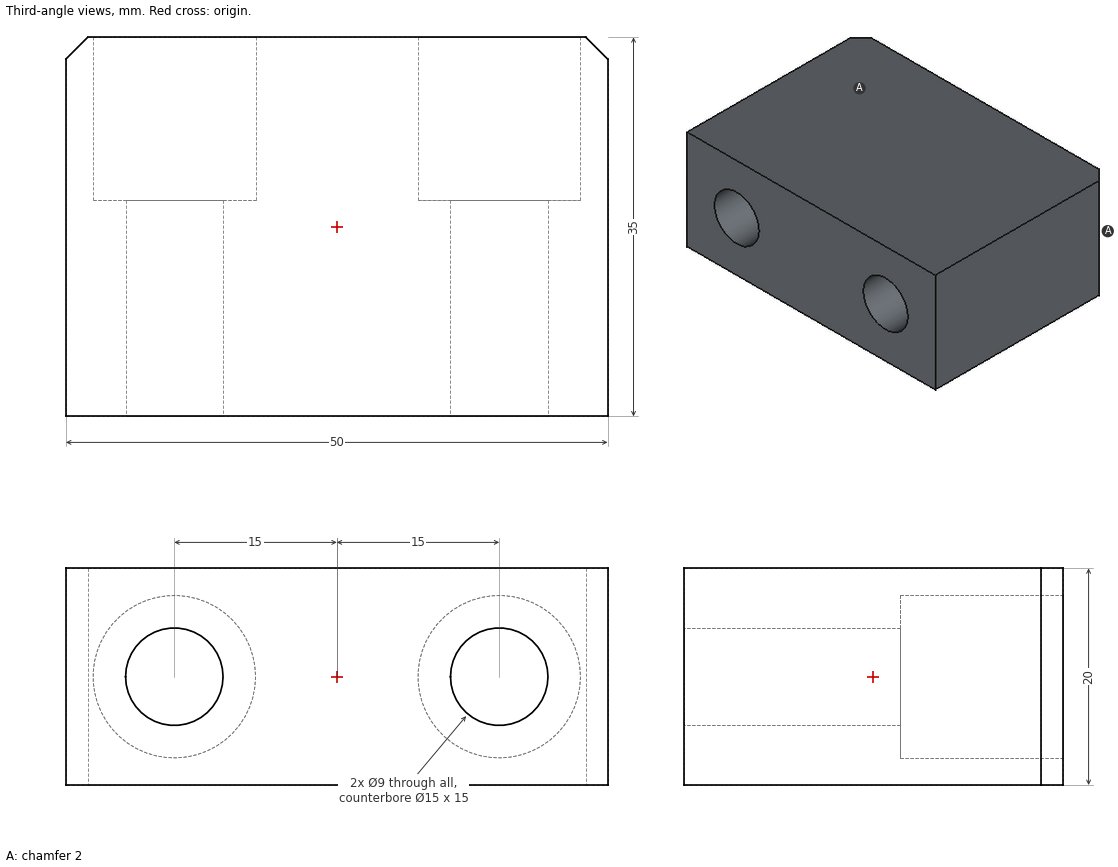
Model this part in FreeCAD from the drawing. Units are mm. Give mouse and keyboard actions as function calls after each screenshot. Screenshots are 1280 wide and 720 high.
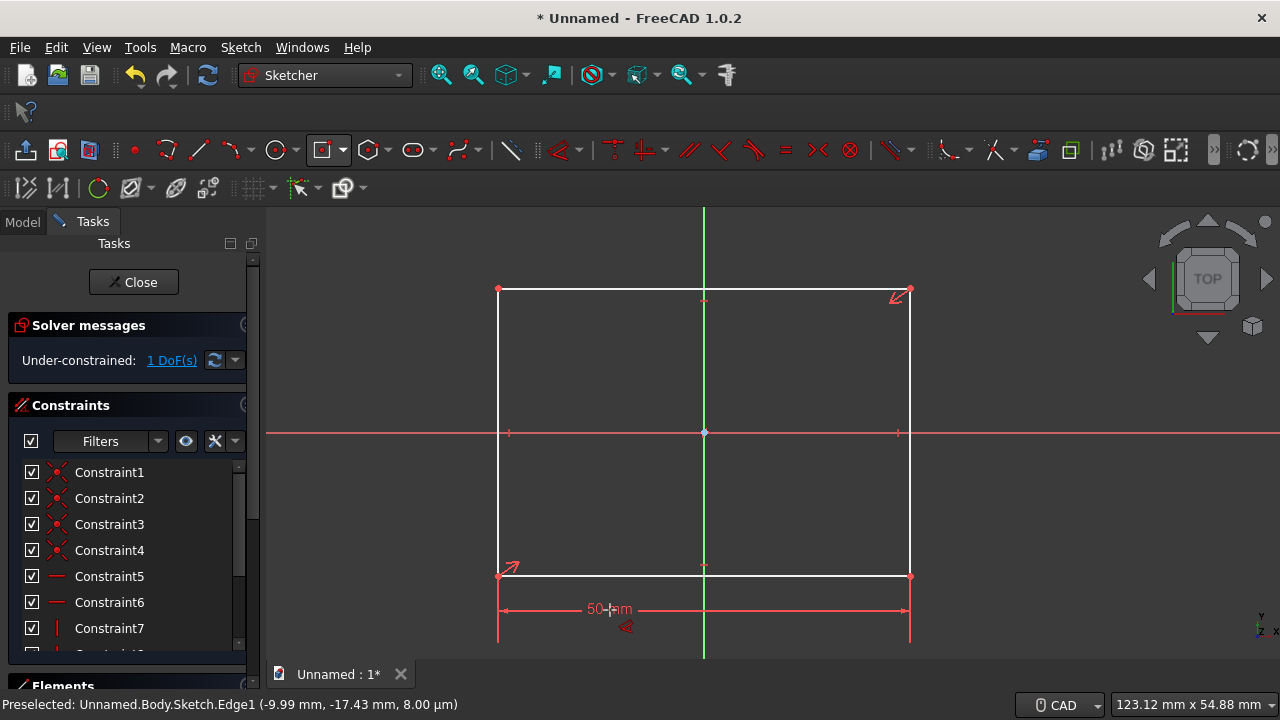
click(910, 490)
click(944, 367)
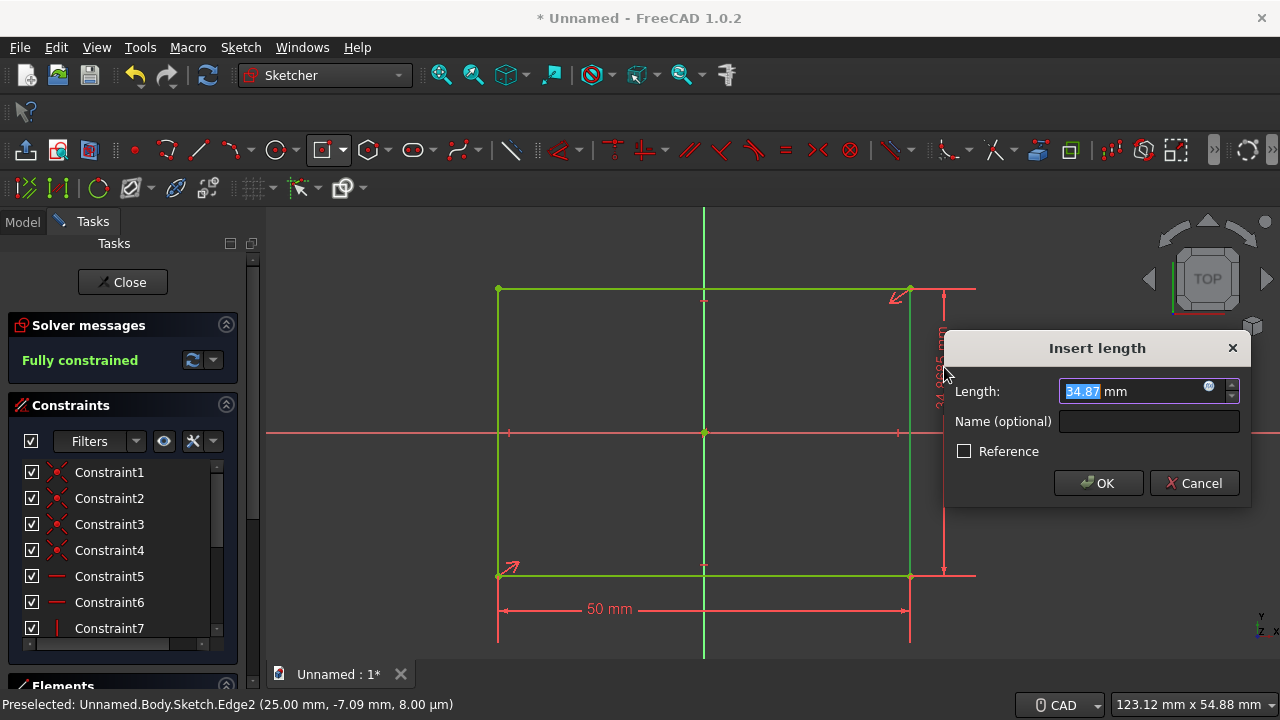
text(35)
key(Return)
key(Escape)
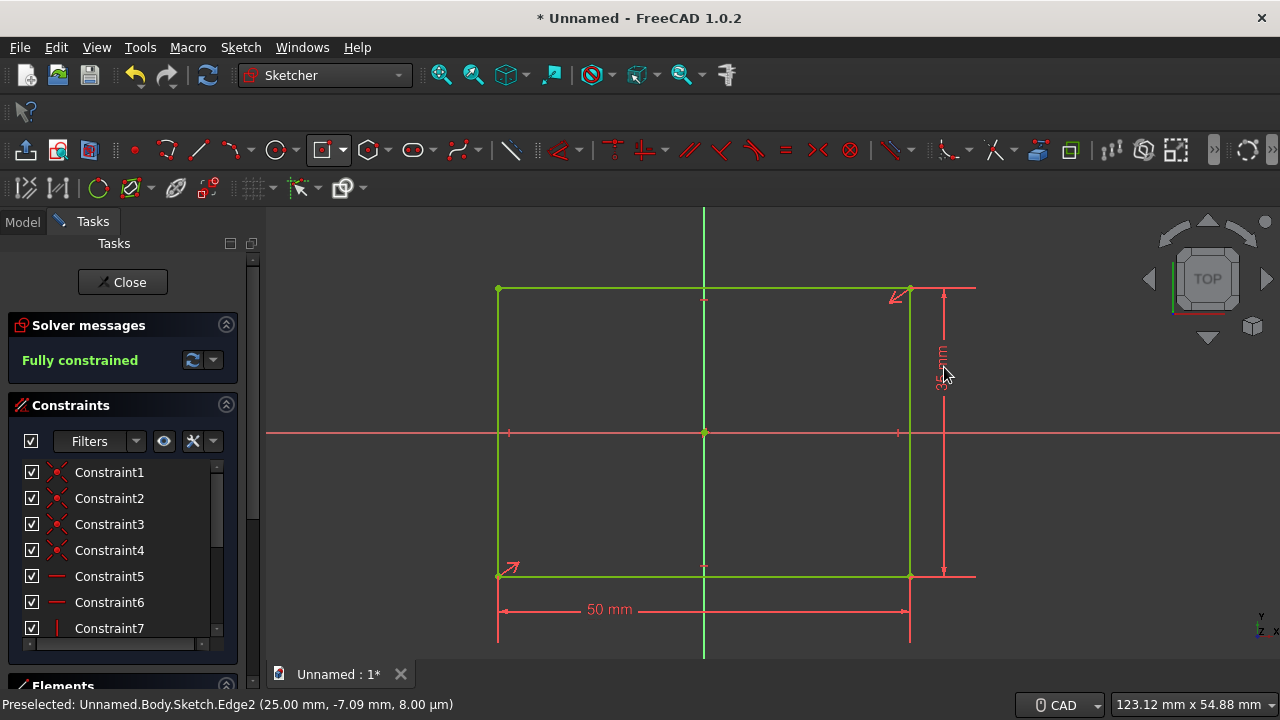
click(123, 282)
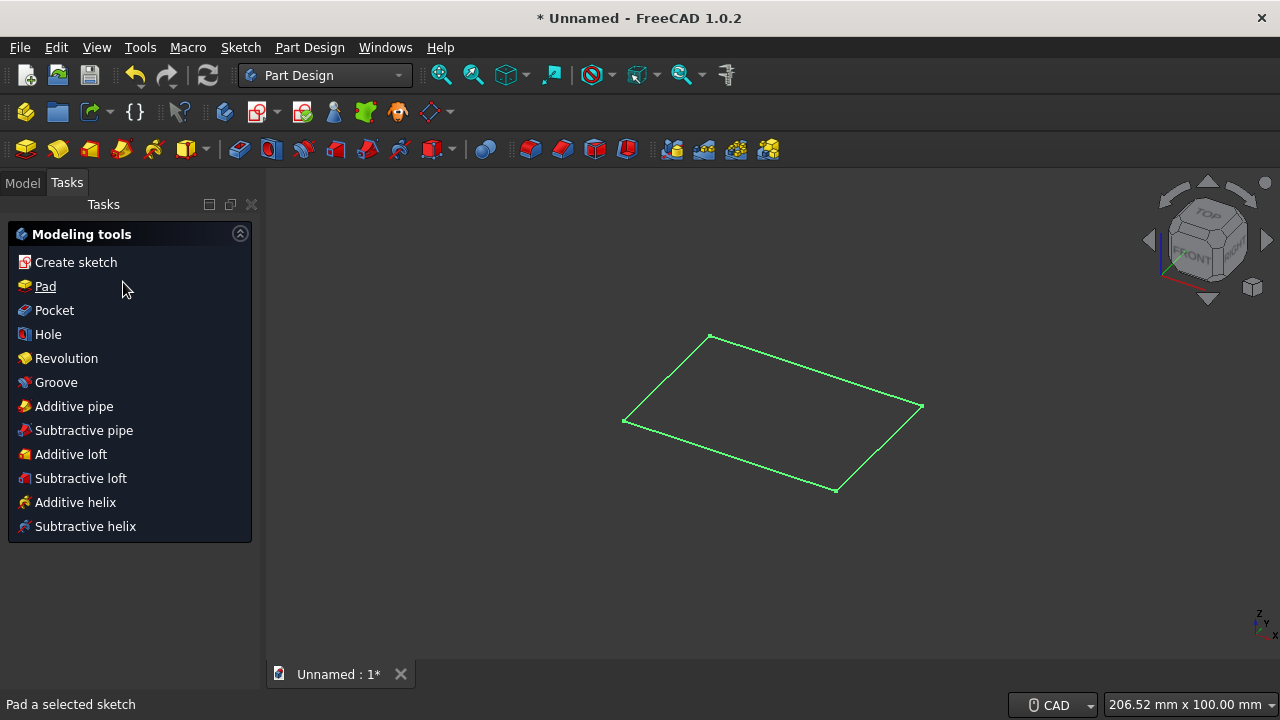
click(26, 150)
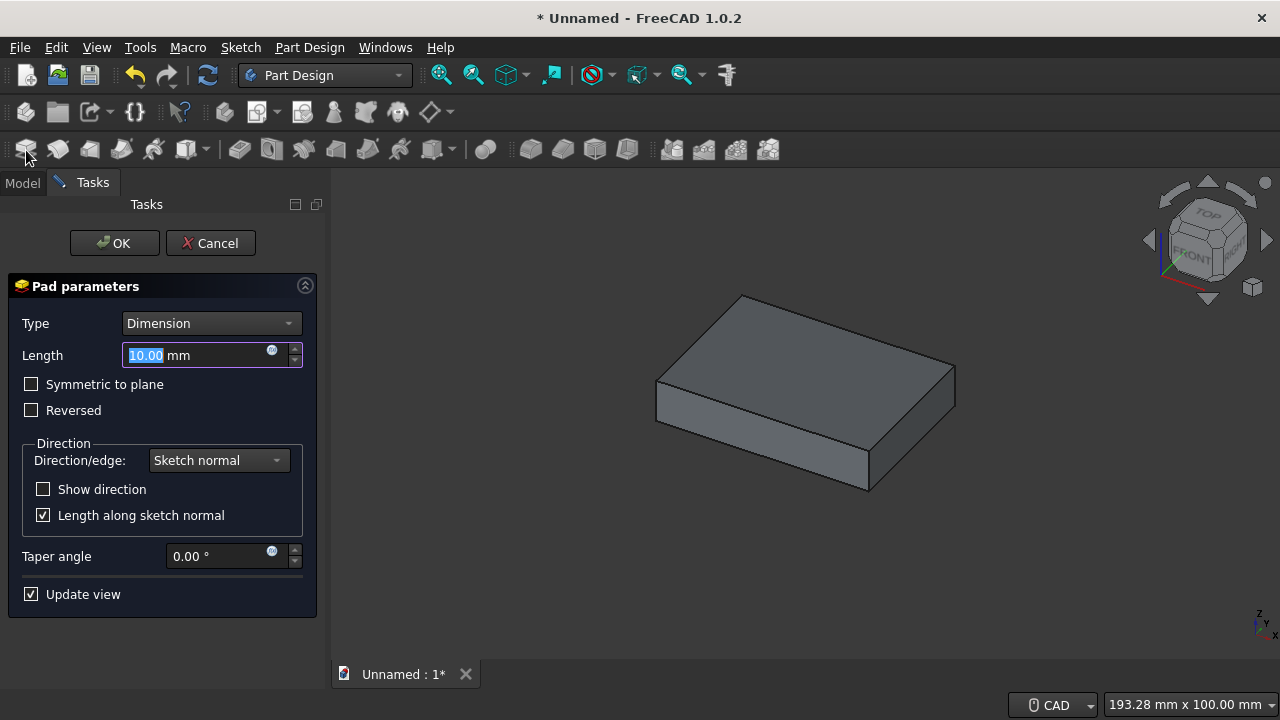
text(20)
key(Tab)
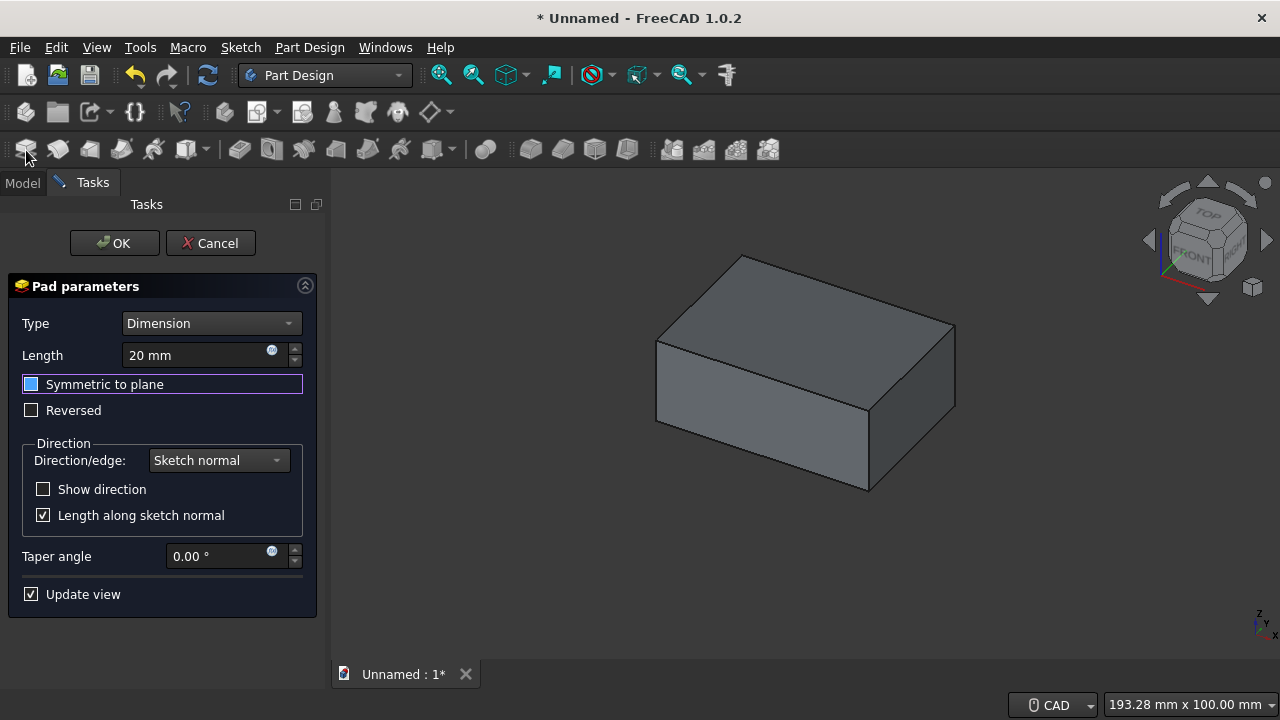
click(30, 384)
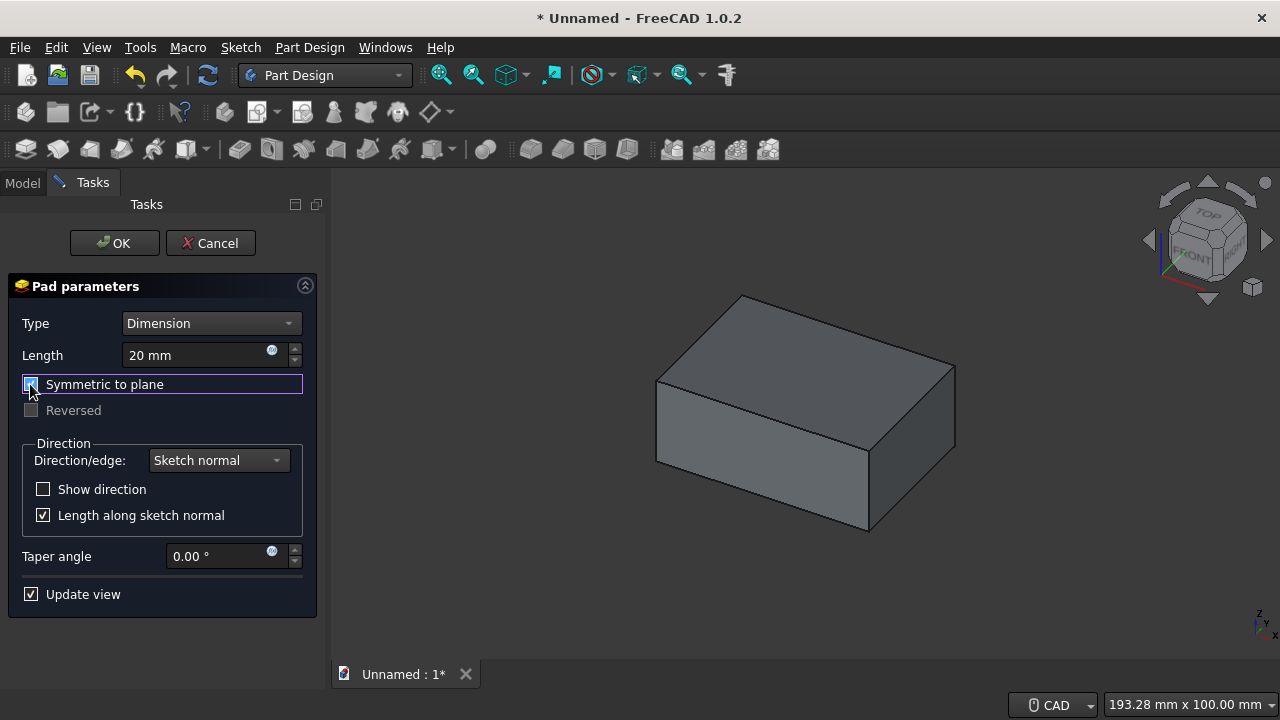
click(115, 243)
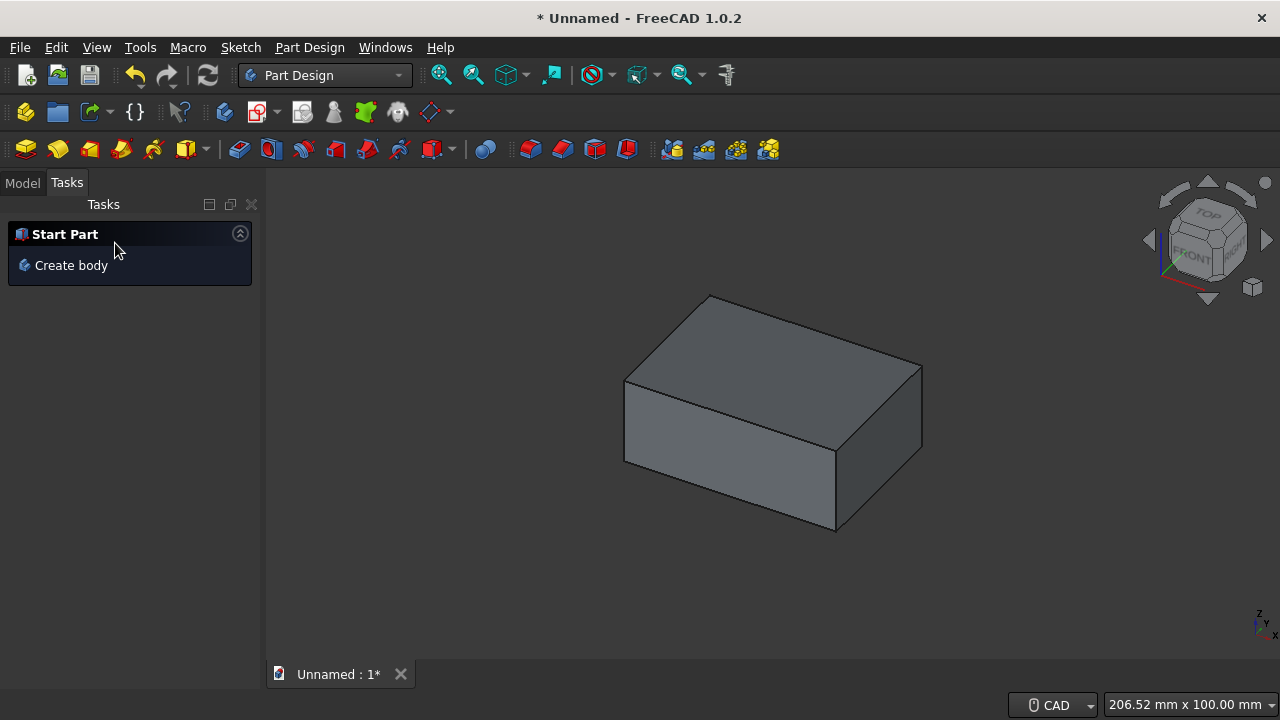
key(4)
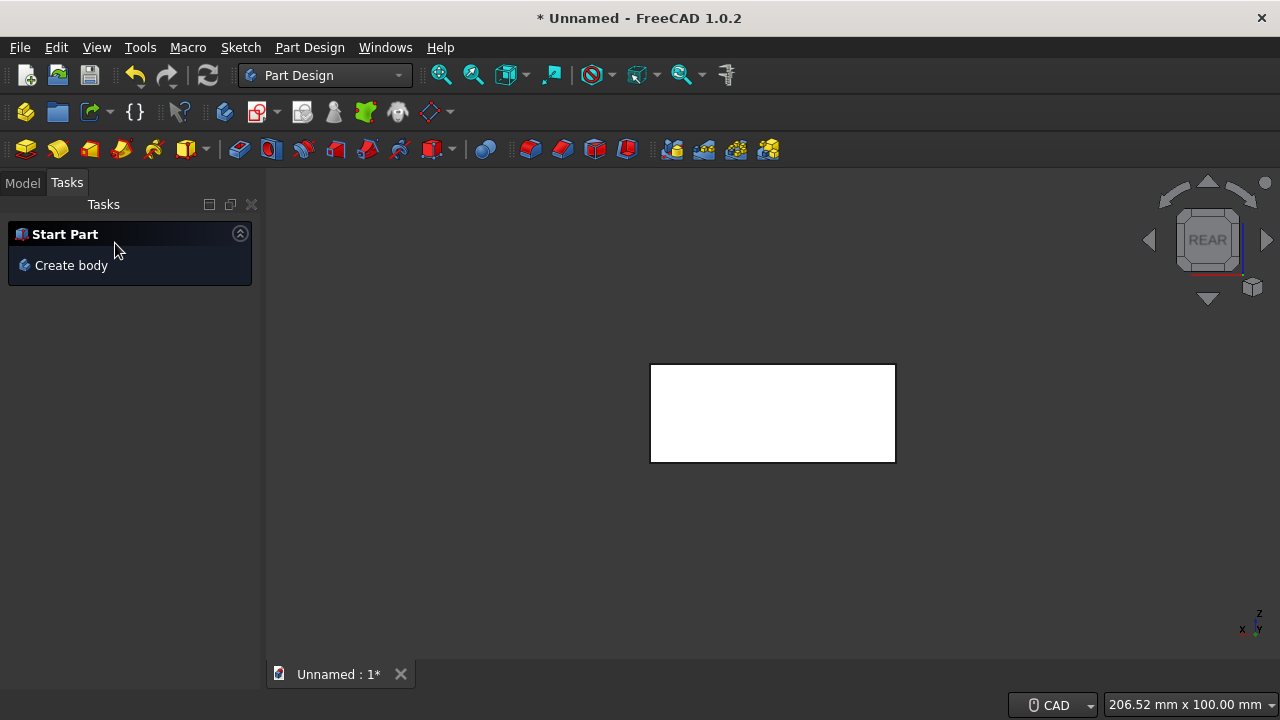
click(442, 76)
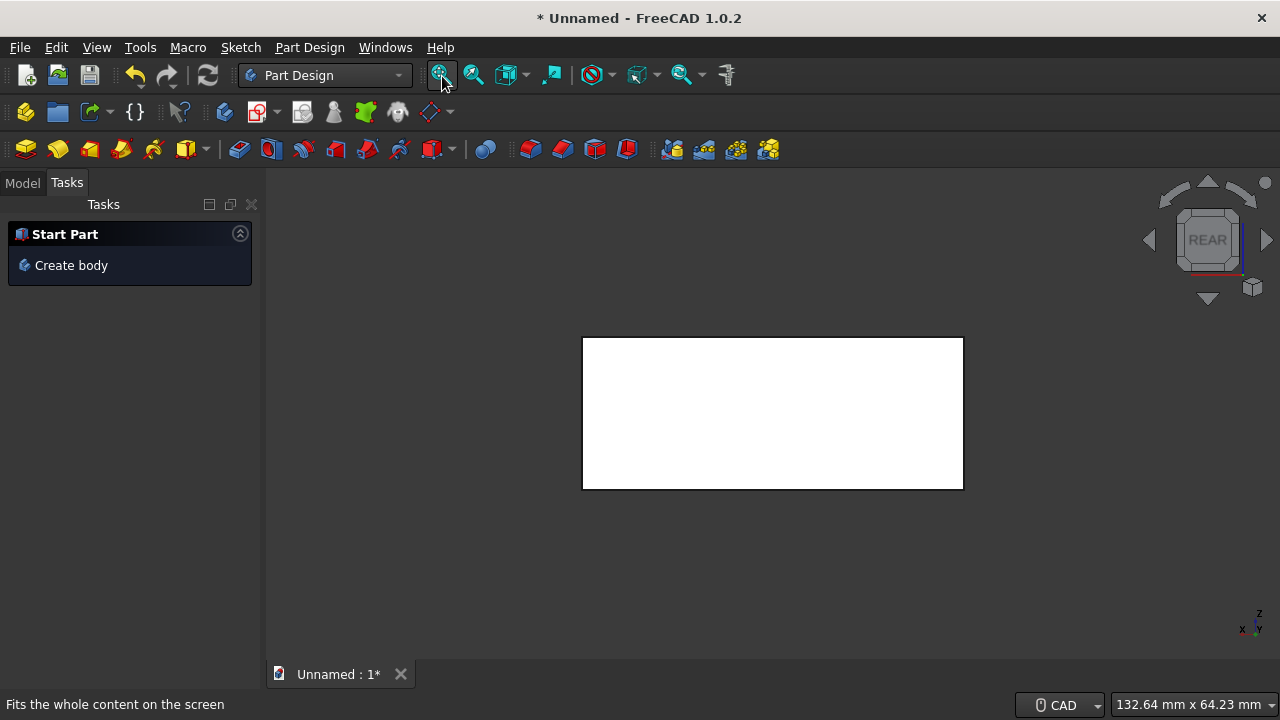
click(664, 413)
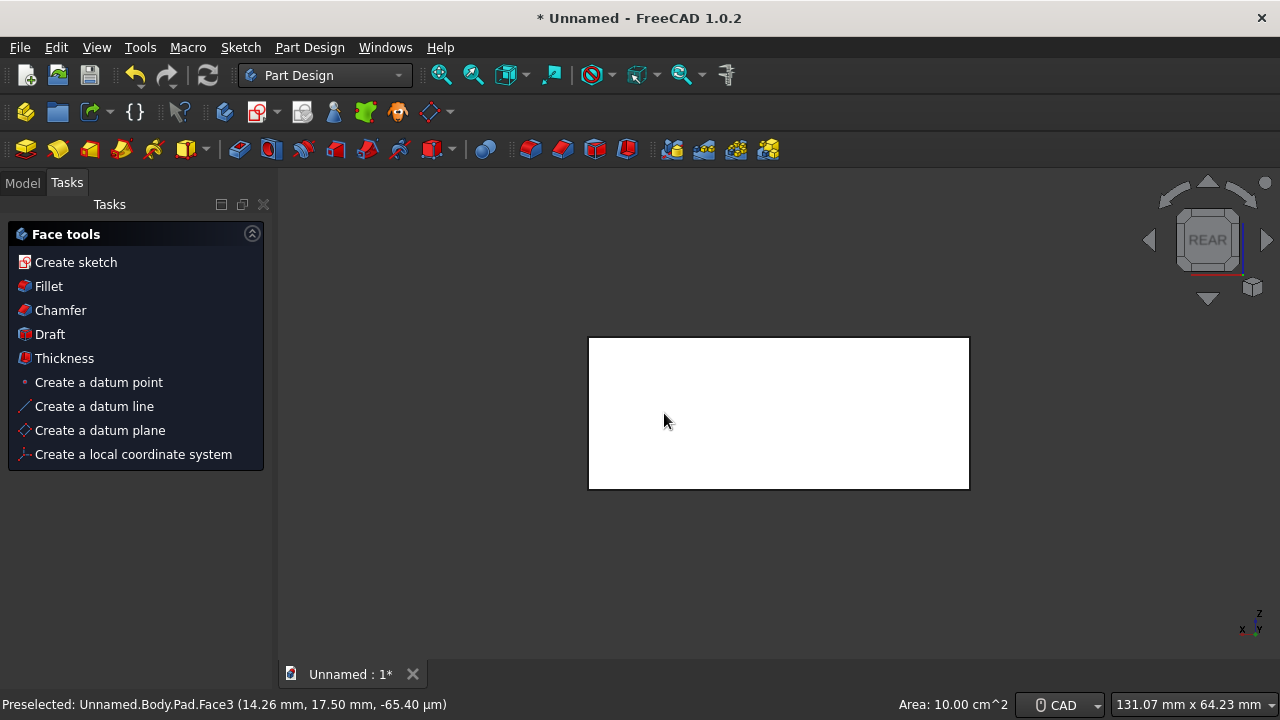
click(258, 112)